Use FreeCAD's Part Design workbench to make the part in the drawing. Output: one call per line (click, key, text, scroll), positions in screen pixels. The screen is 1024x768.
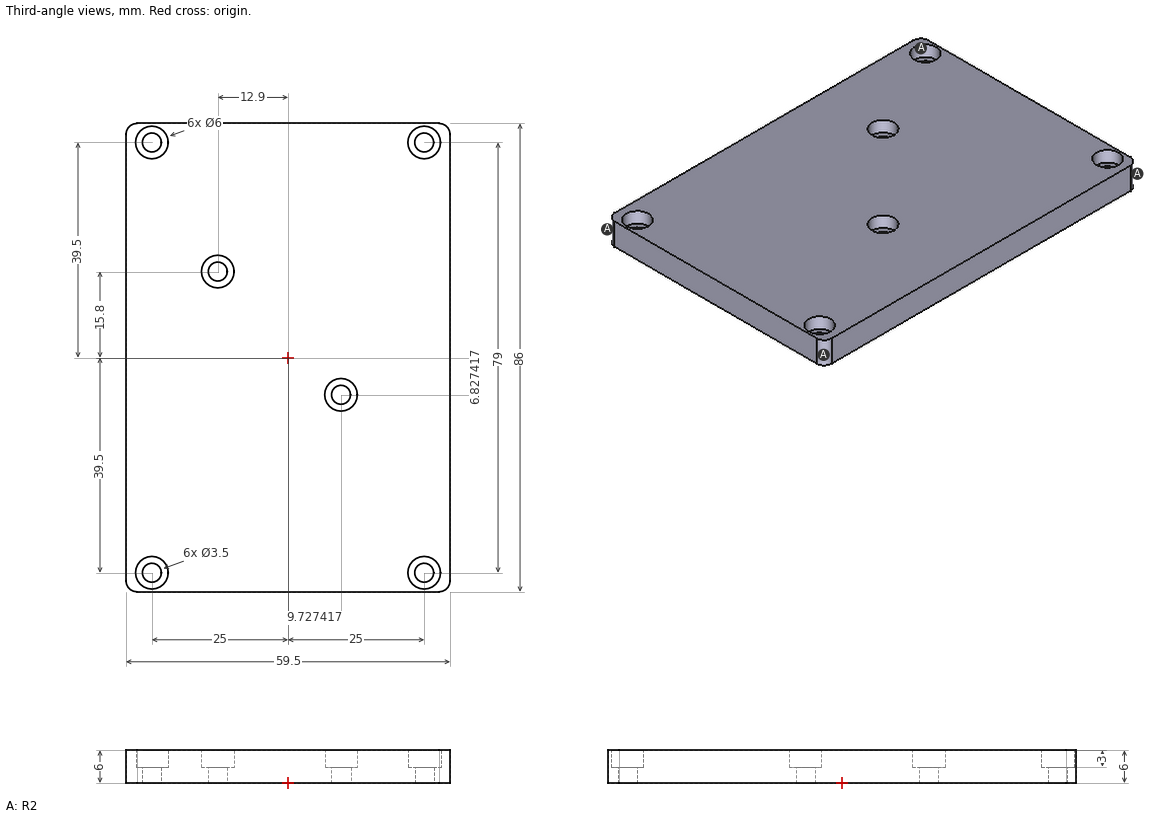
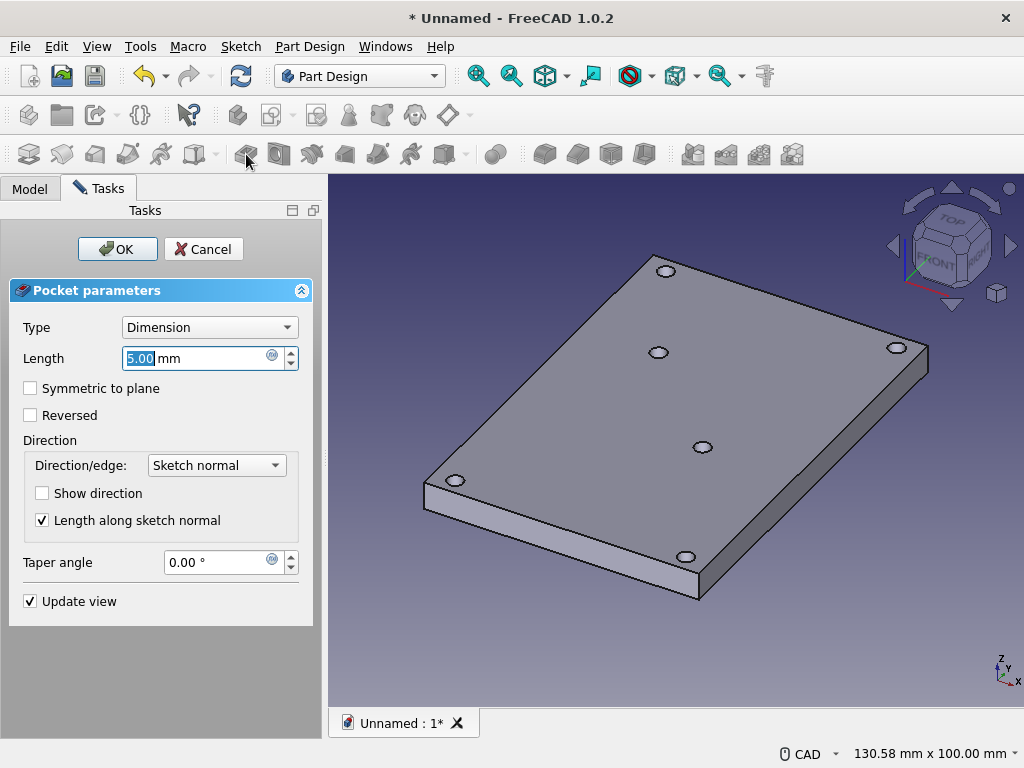
text(6)
key(Tab)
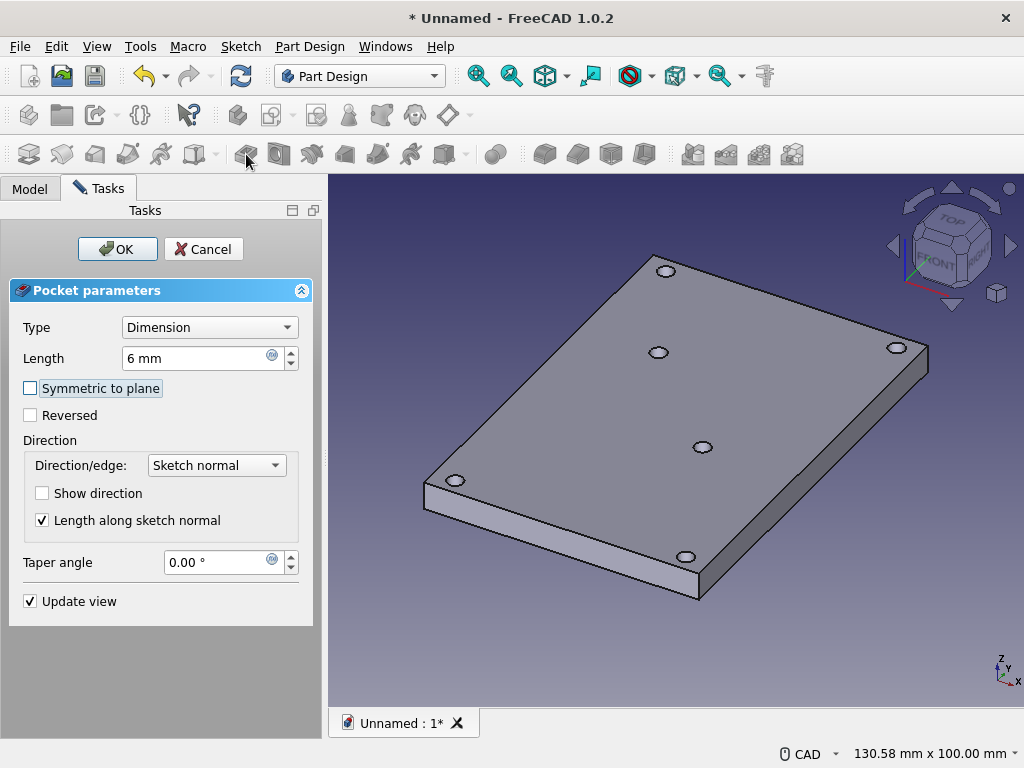
click(118, 249)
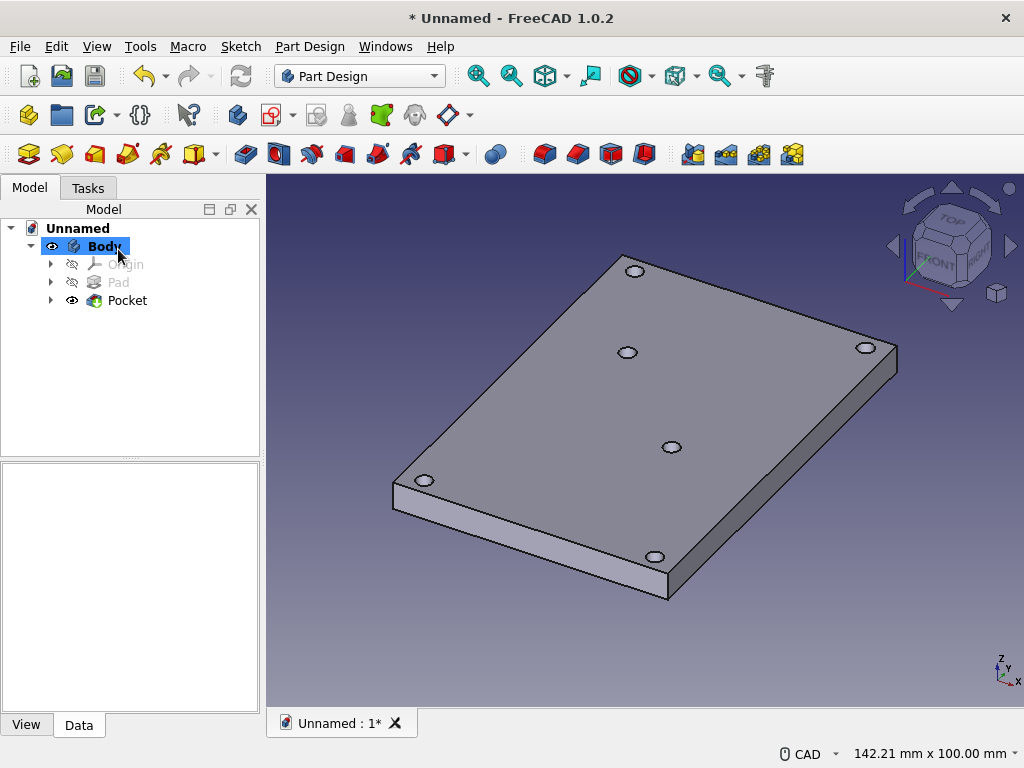
click(750, 361)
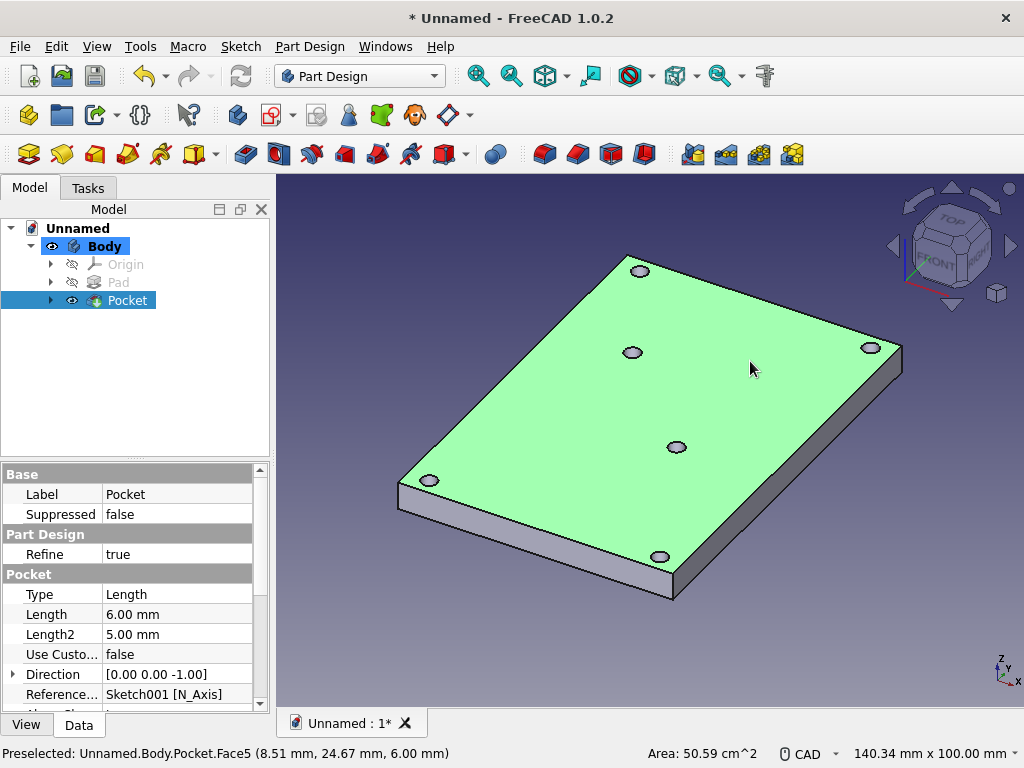
click(270, 116)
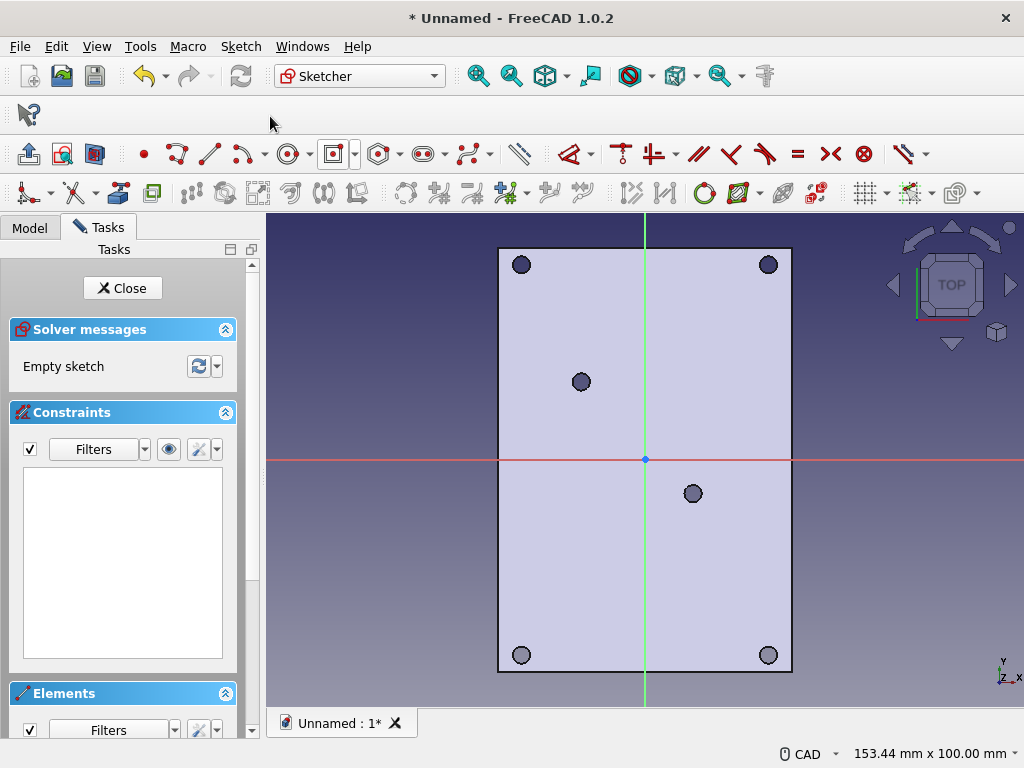
scroll(437, 460, down, 2)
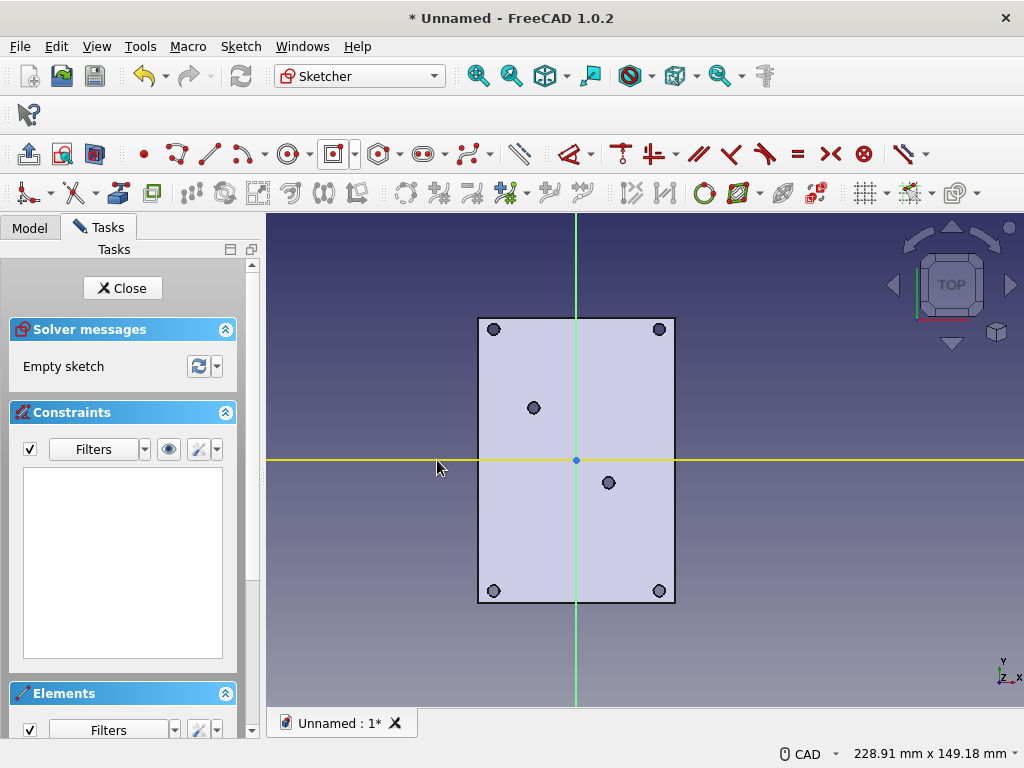
key(g)
key(c)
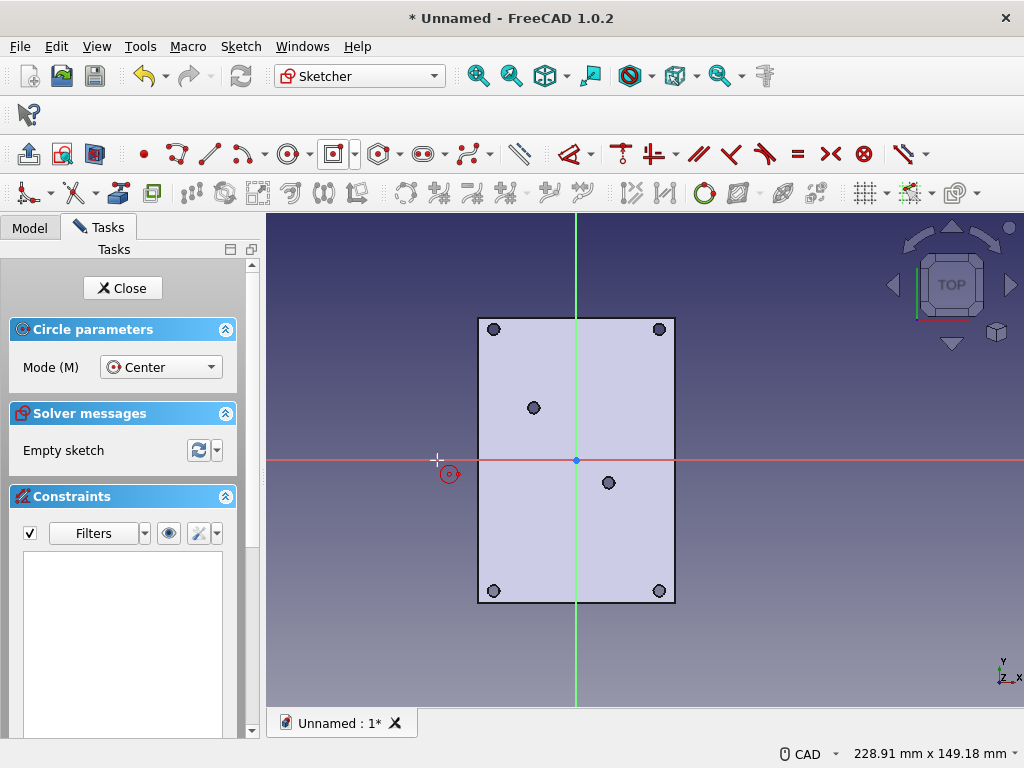
scroll(494, 329, up, 5)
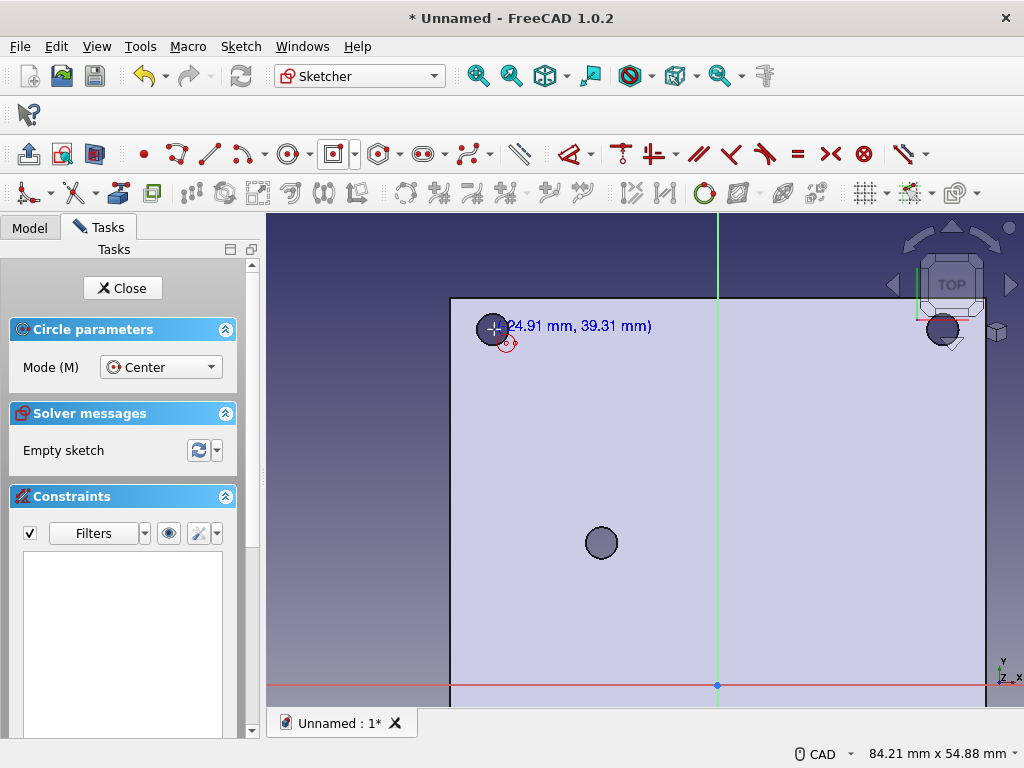
click(493, 330)
click(512, 310)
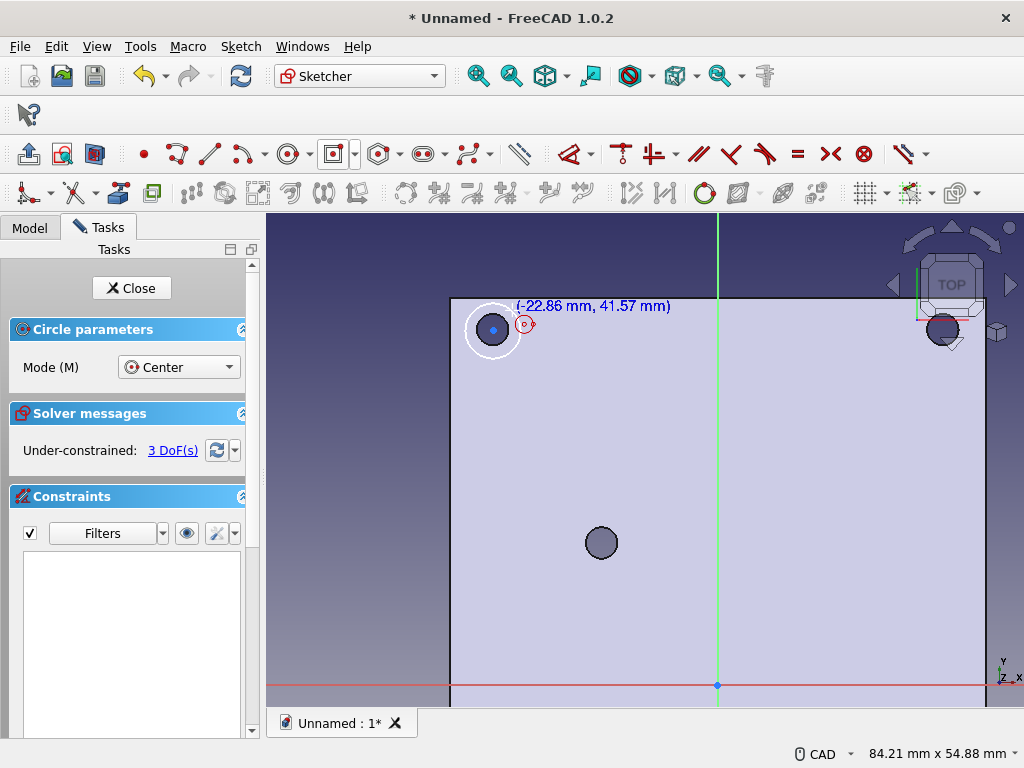
scroll(494, 329, down, 5)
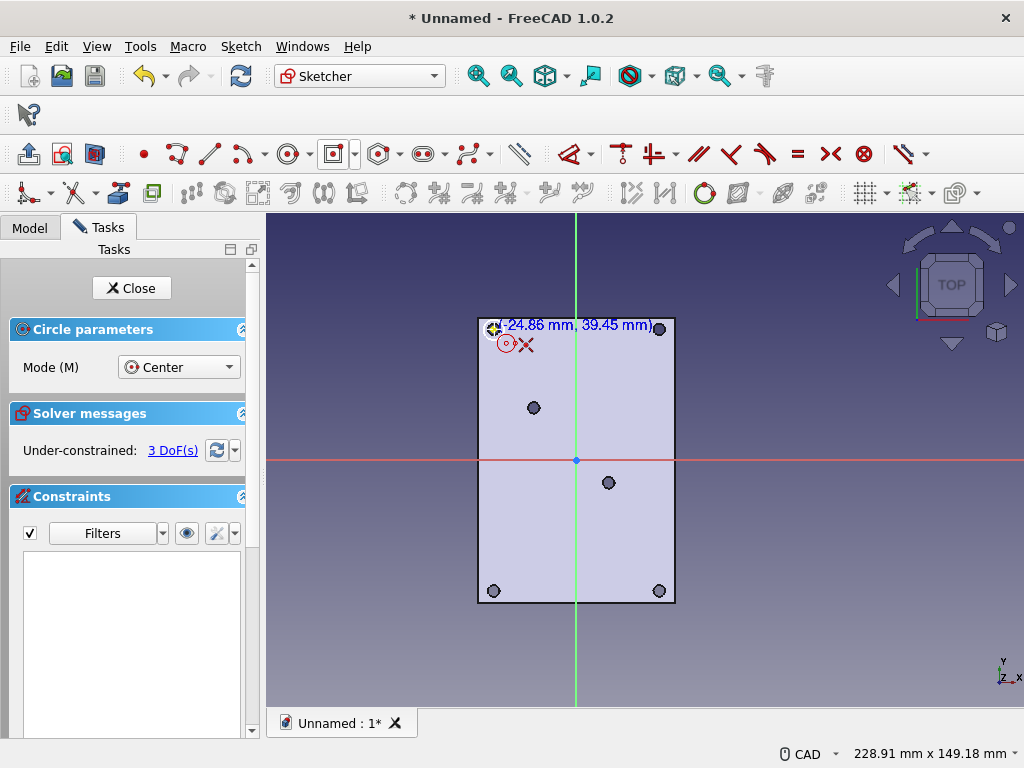
scroll(659, 329, up, 5)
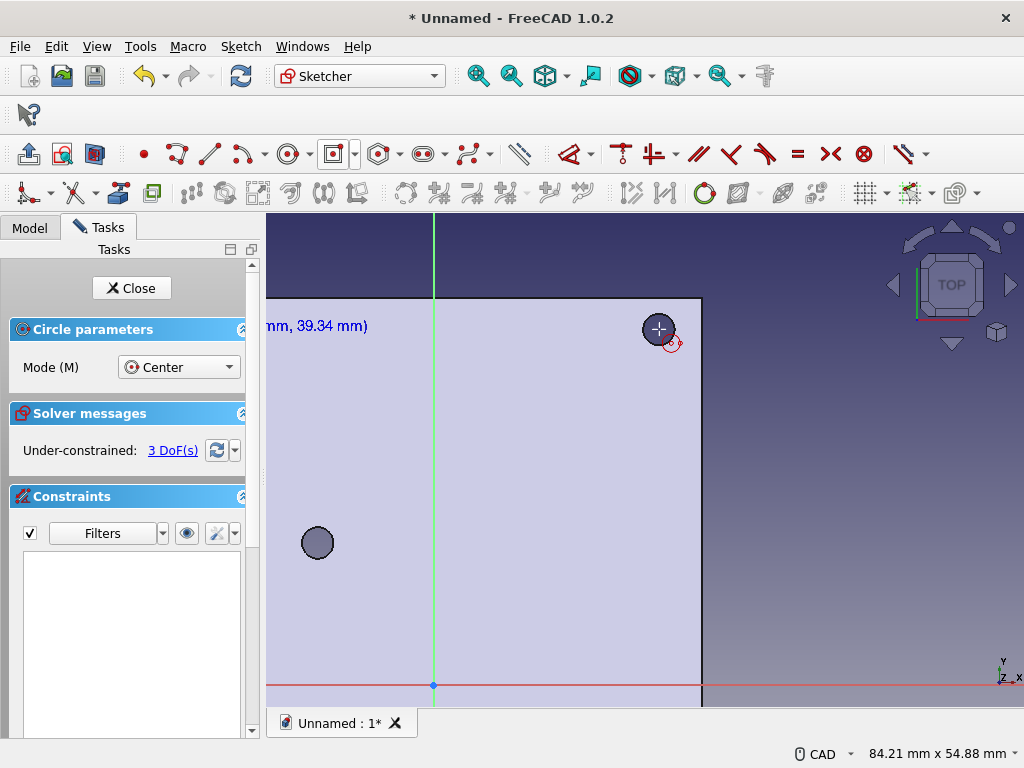
click(659, 330)
click(678, 310)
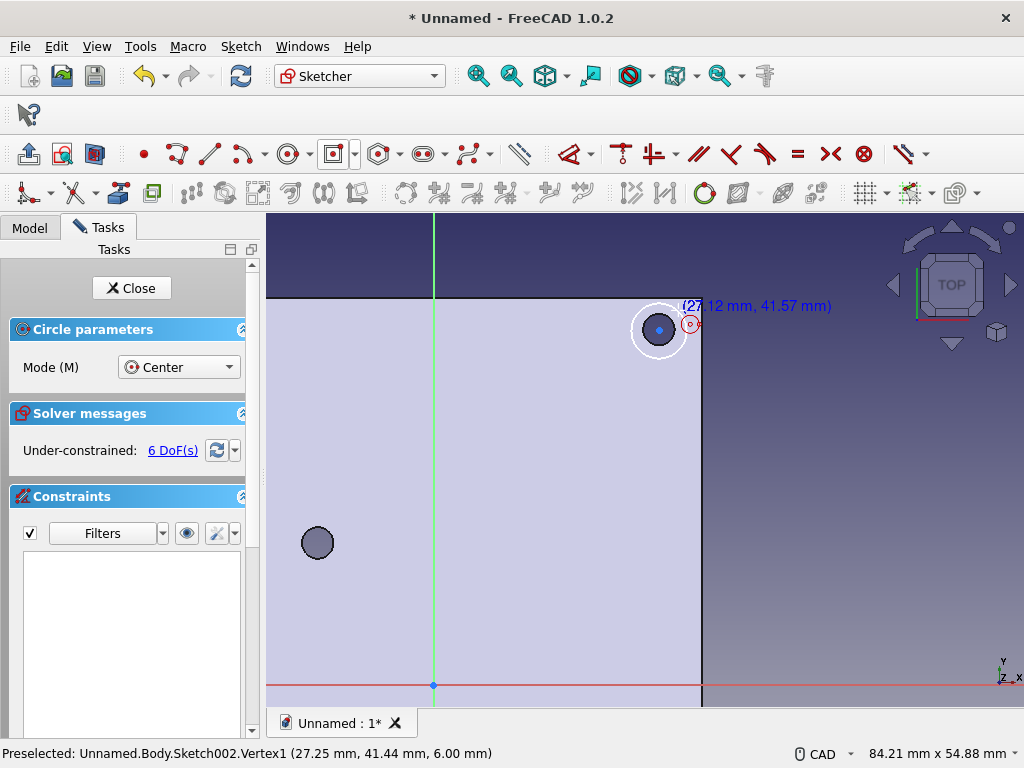
click(318, 543)
click(337, 524)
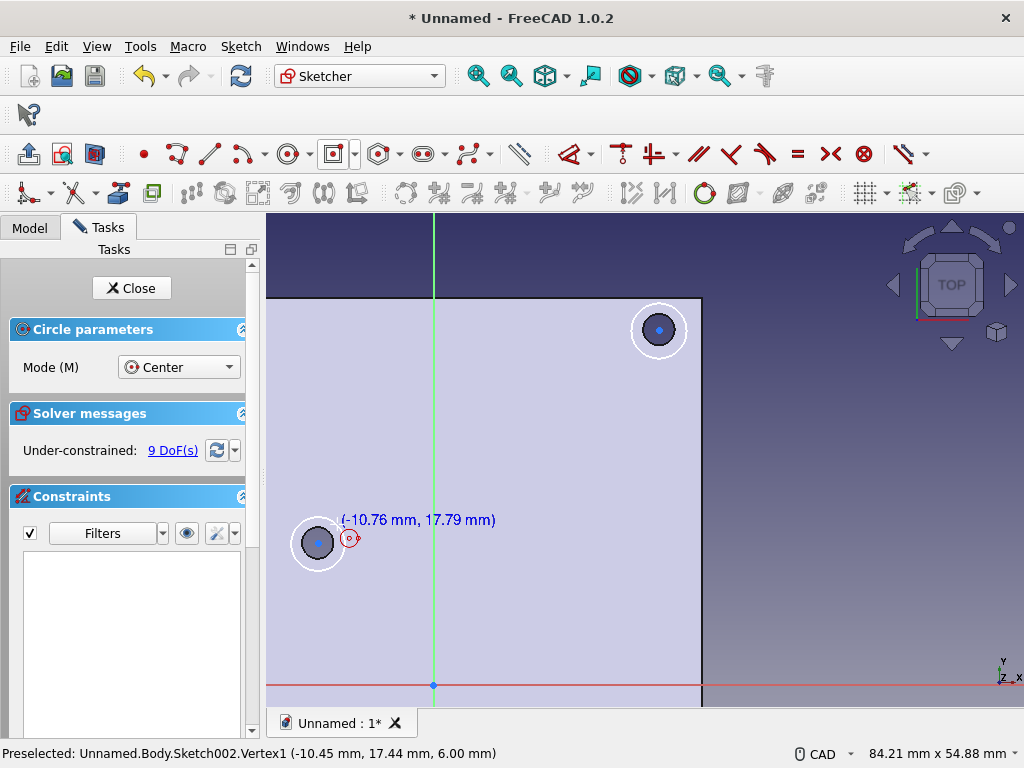
scroll(660, 329, down, 5)